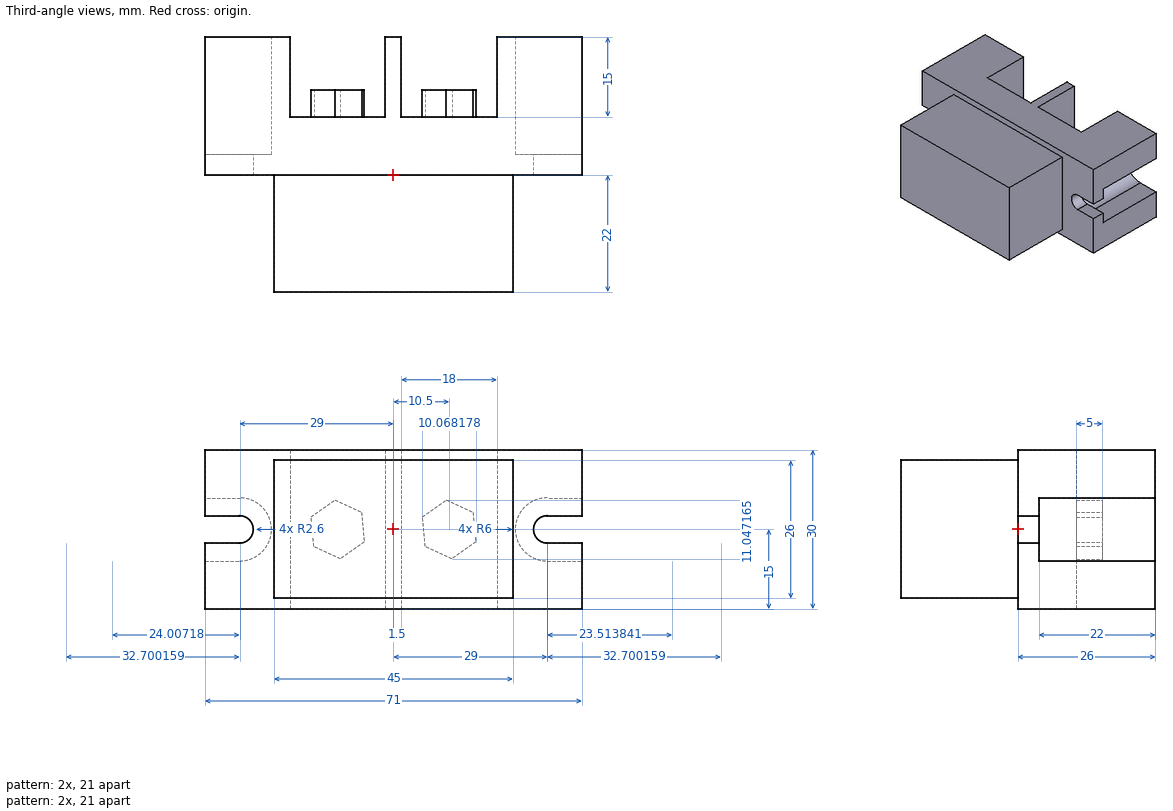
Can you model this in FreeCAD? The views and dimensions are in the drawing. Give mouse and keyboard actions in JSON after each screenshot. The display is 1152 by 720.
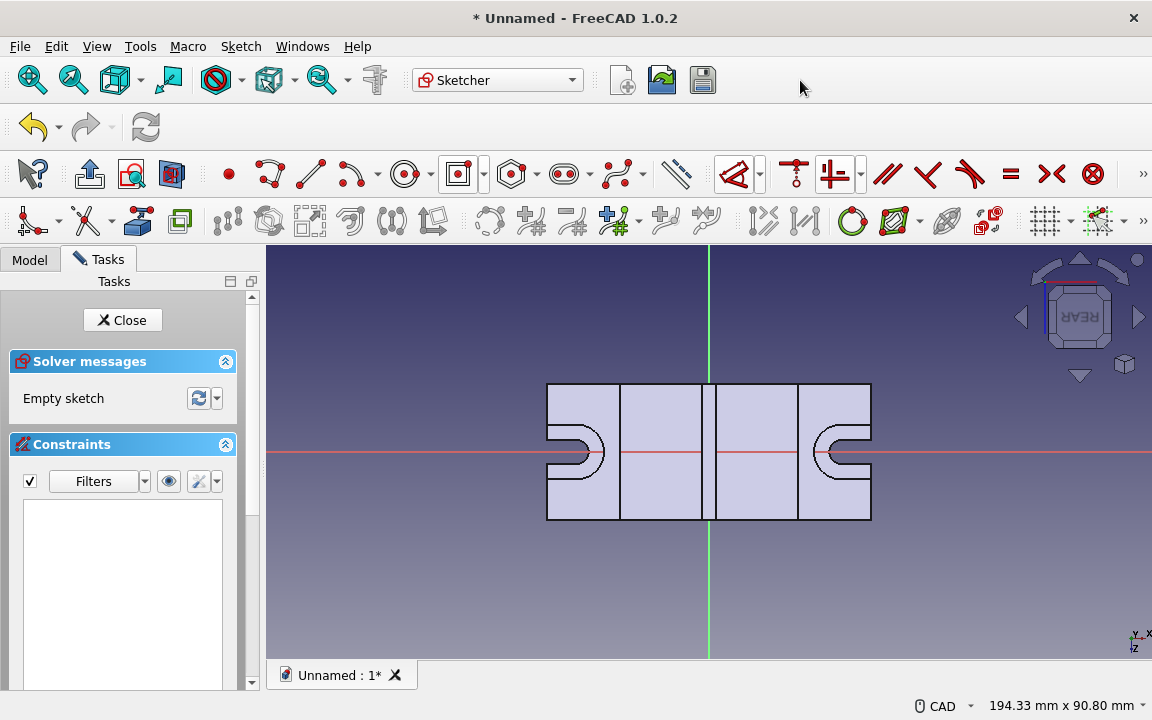
{"action": "scroll", "coordinate": [771, 452], "scroll_direction": "up", "scroll_amount": 8}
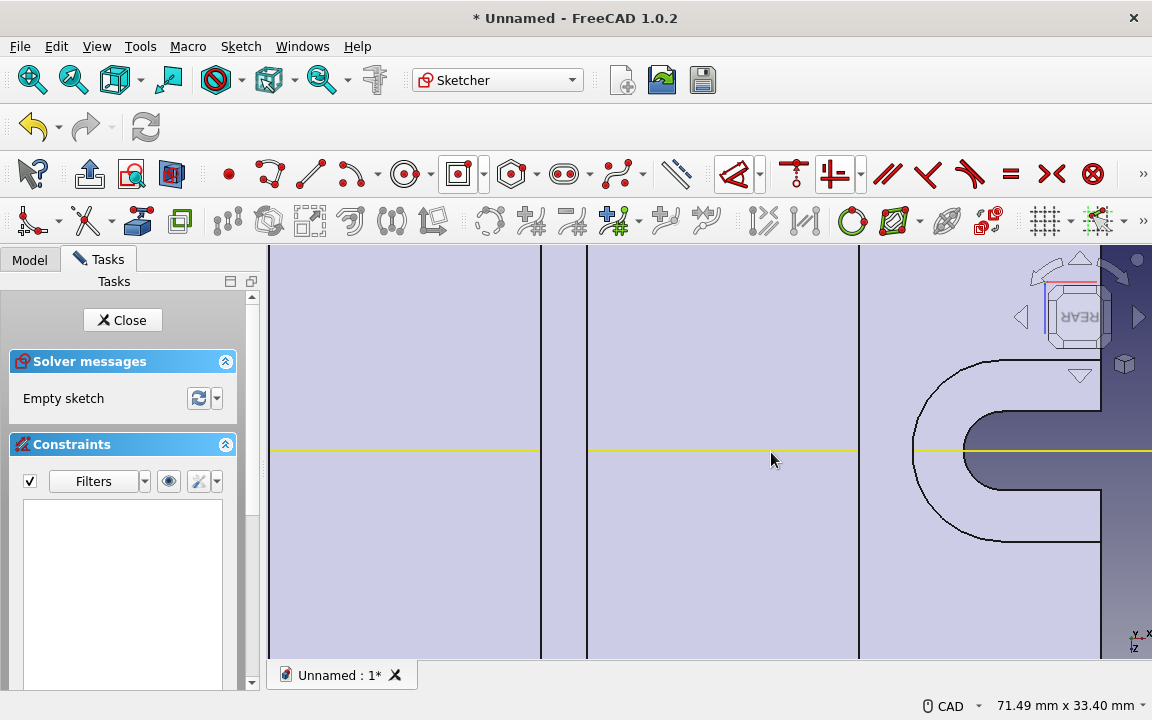
{"action": "left_click", "coordinate": [510, 174]}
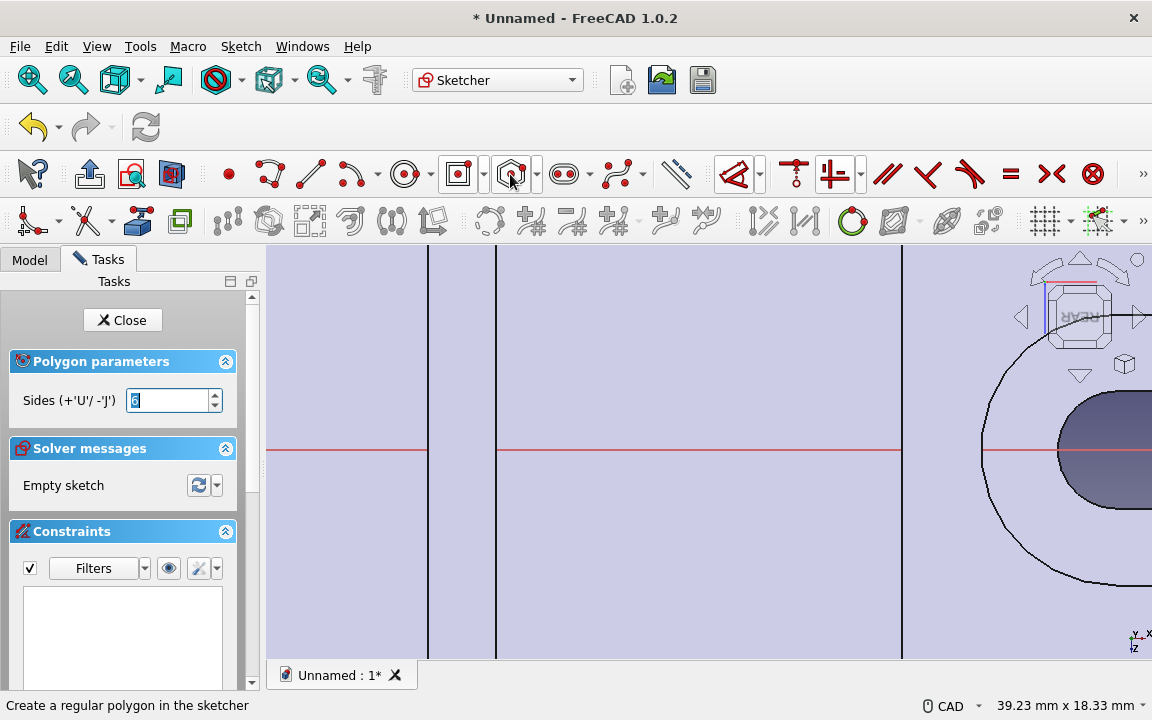
{"action": "left_click", "coordinate": [699, 450]}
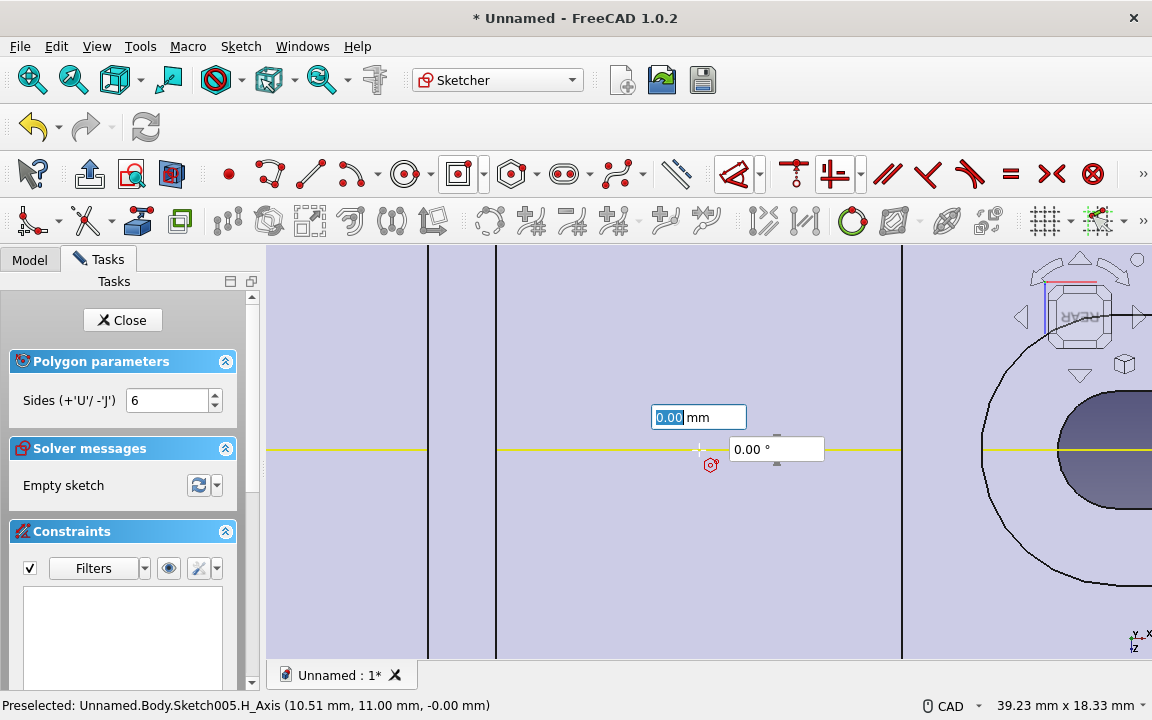
{"action": "left_click", "coordinate": [710, 325]}
{"action": "right_click", "coordinate": [710, 325]}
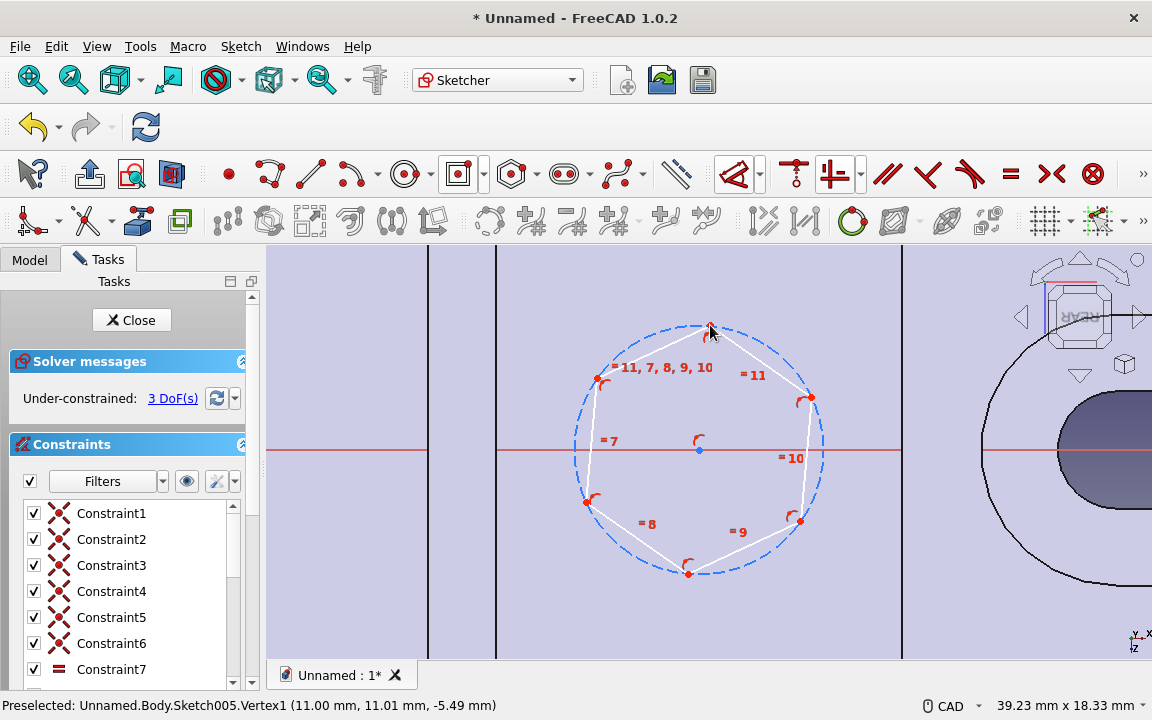
{"action": "left_click", "coordinate": [699, 450]}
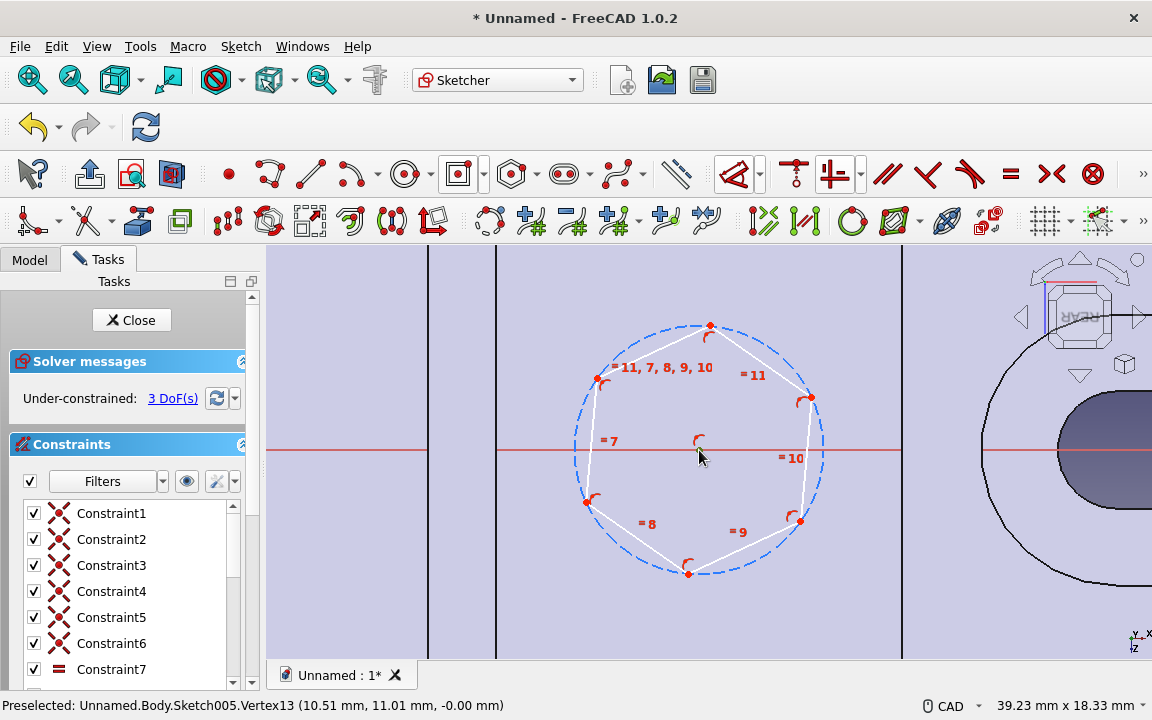
{"action": "left_click", "coordinate": [760, 174]}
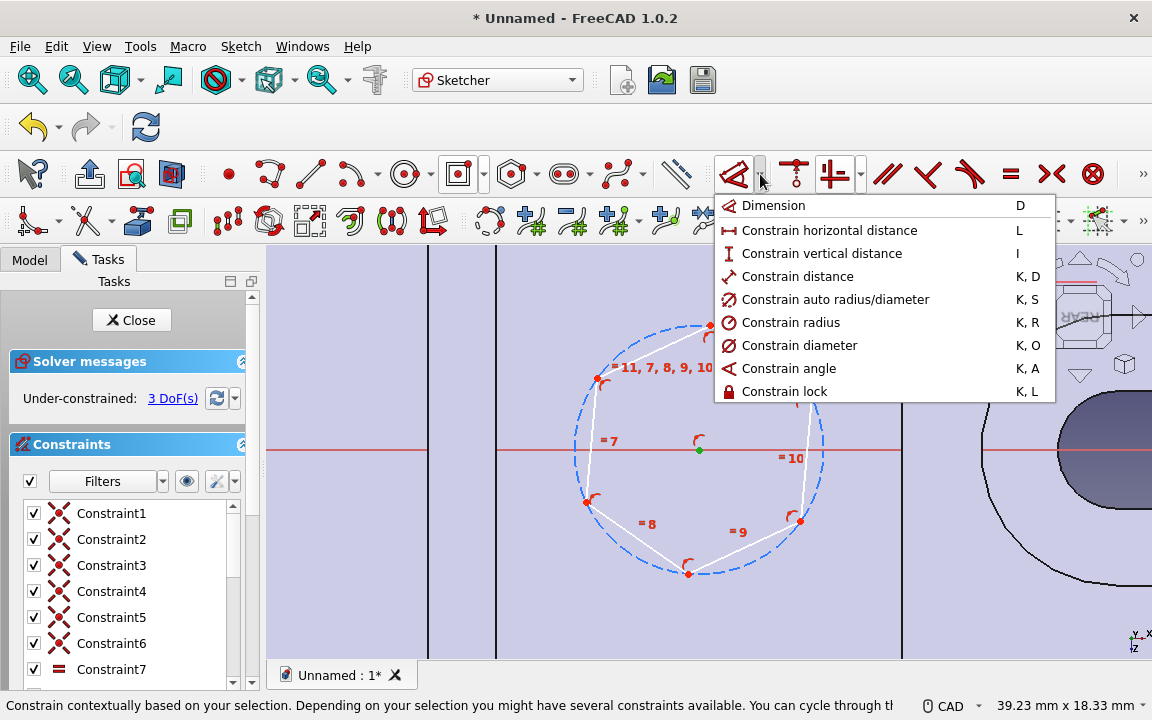
{"action": "left_click", "coordinate": [885, 230]}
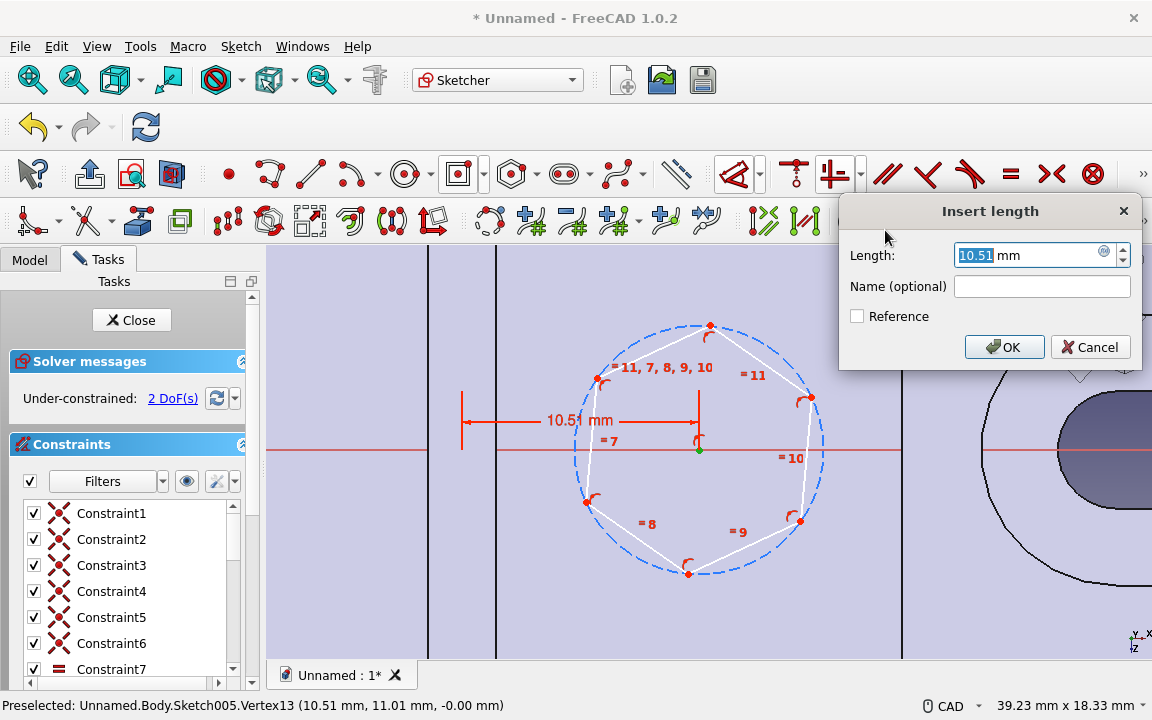
{"action": "type", "text": "10.5"}
{"action": "key", "text": "Return"}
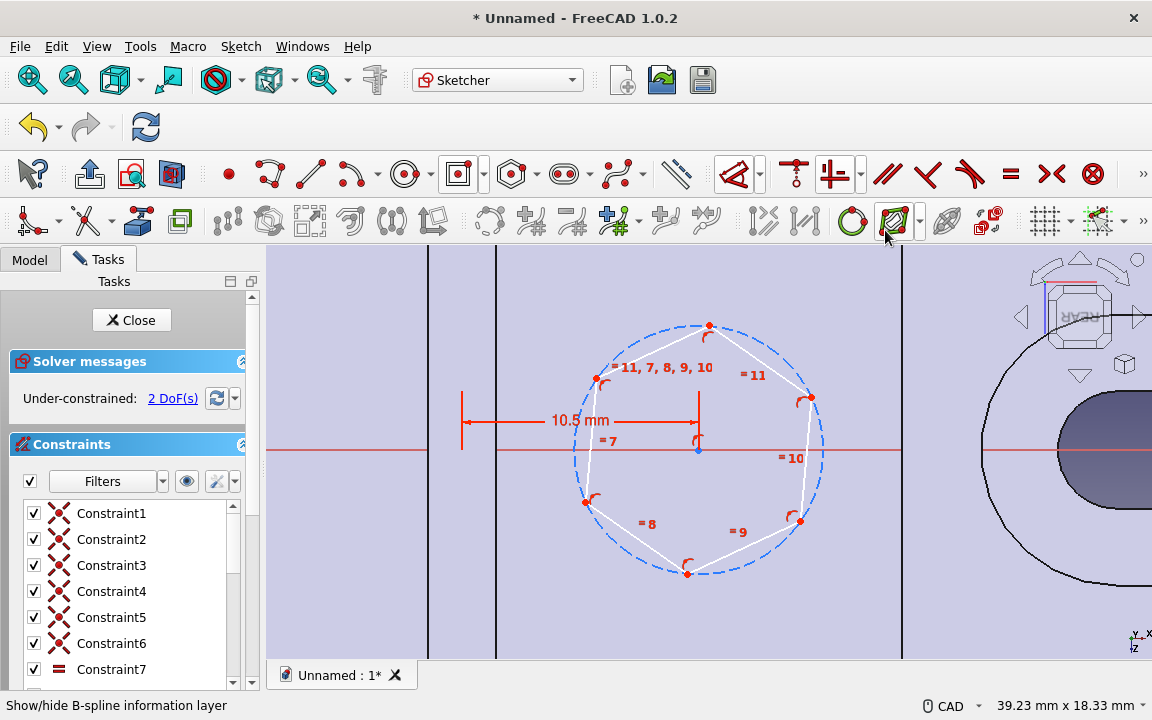
{"action": "left_click", "coordinate": [586, 503]}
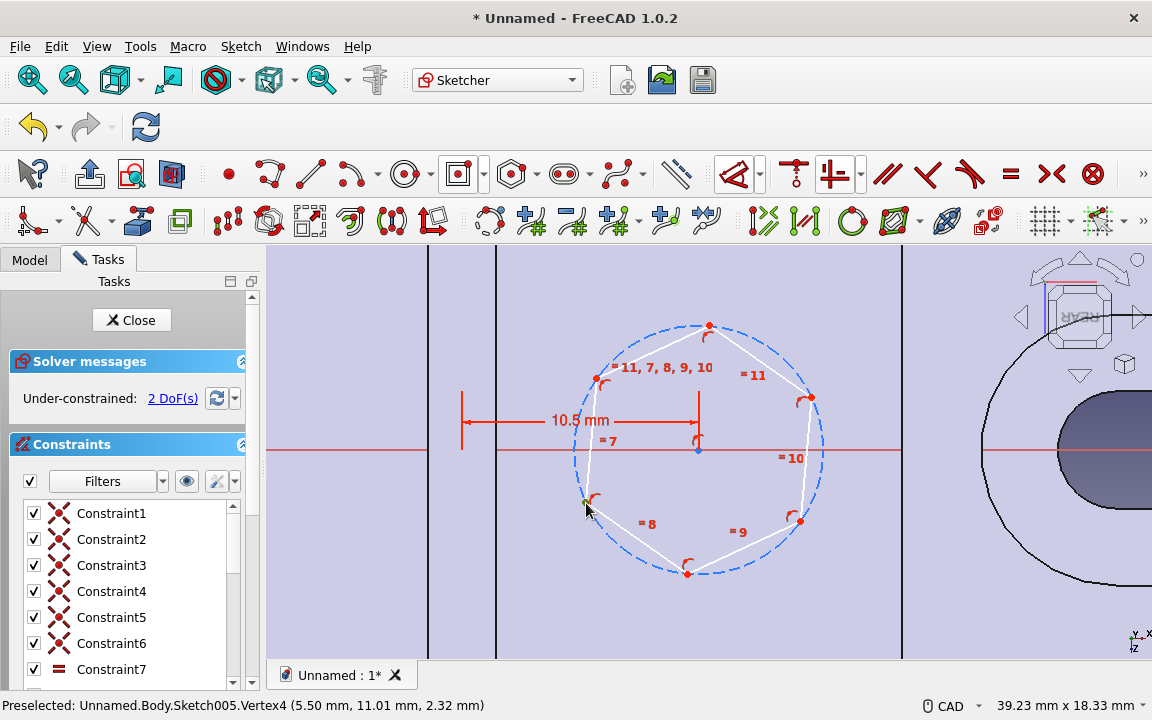
{"action": "left_click", "coordinate": [812, 398]}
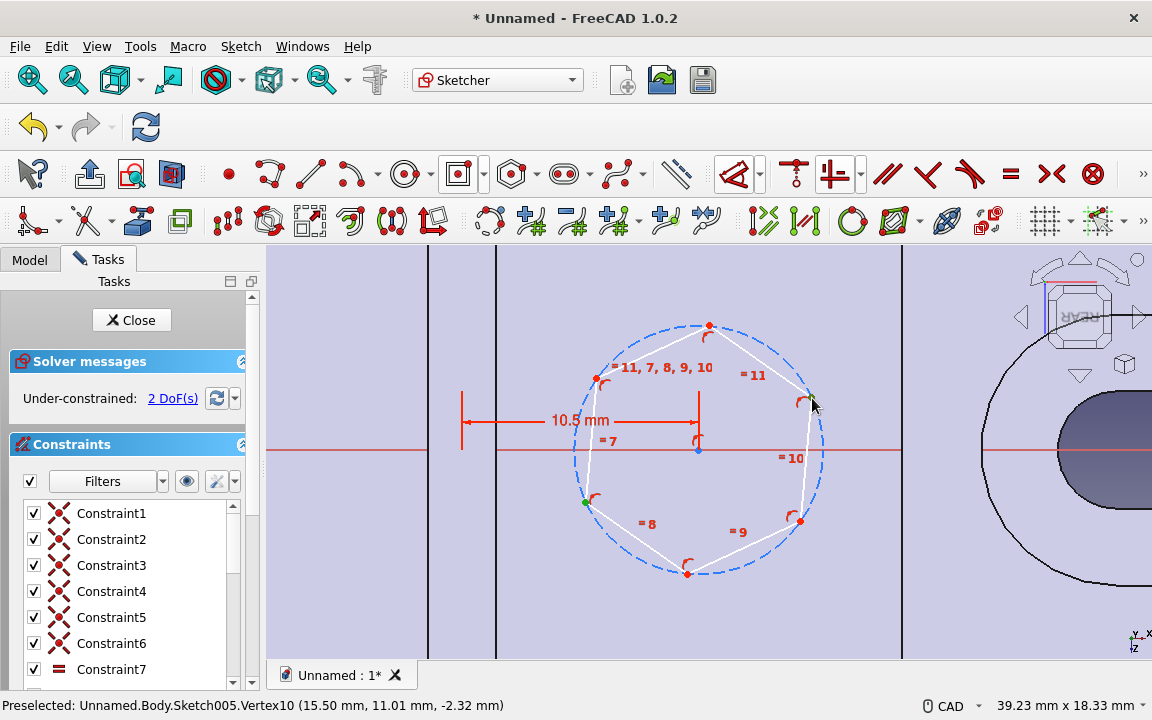
{"action": "left_click", "coordinate": [760, 174]}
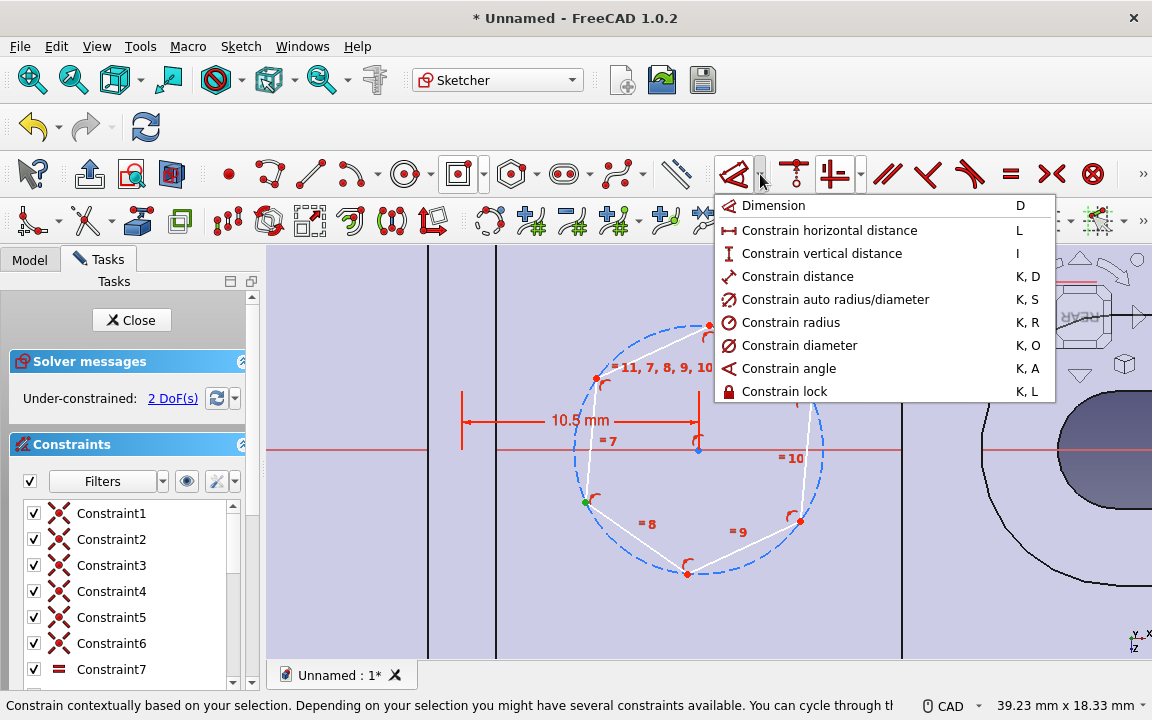
{"action": "left_click", "coordinate": [885, 230]}